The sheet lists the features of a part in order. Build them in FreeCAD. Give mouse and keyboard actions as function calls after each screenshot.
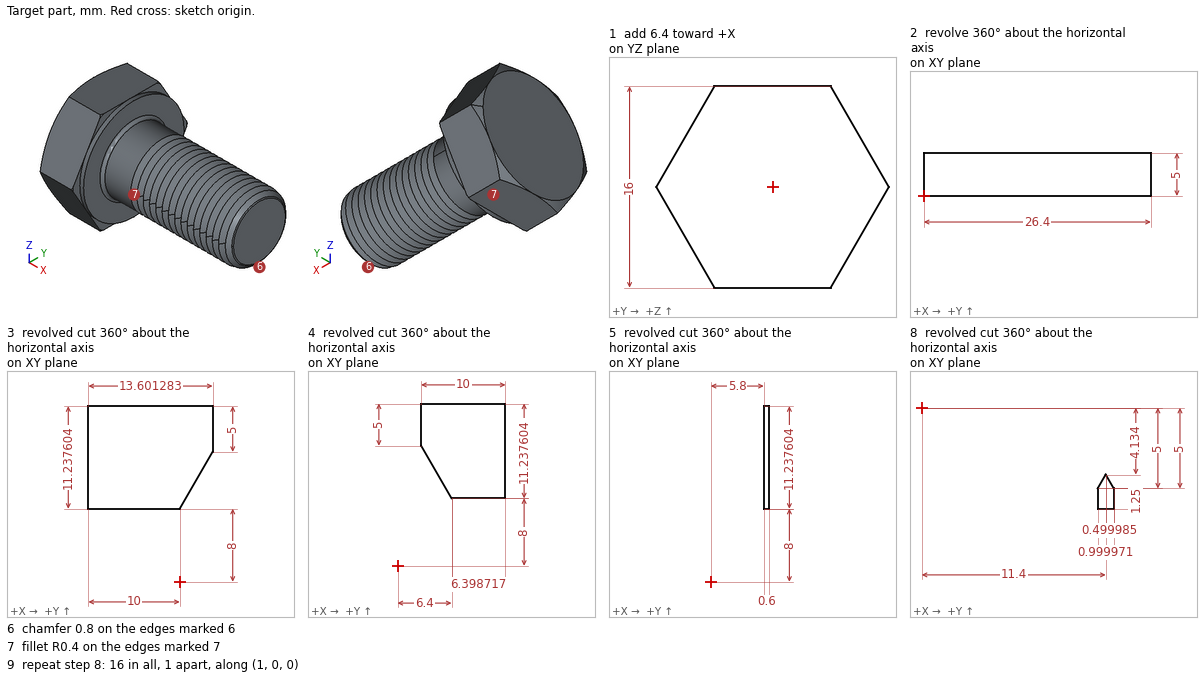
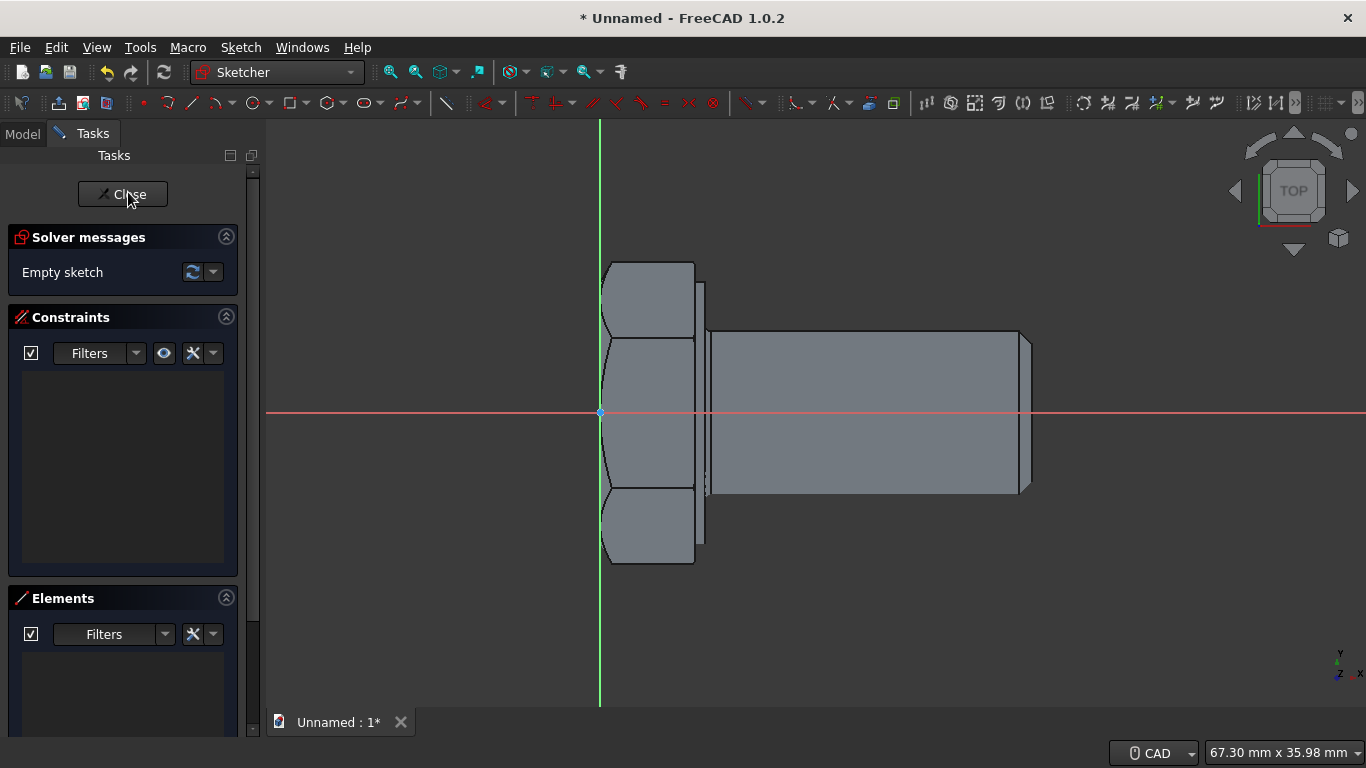
scroll(790, 506, up, 12)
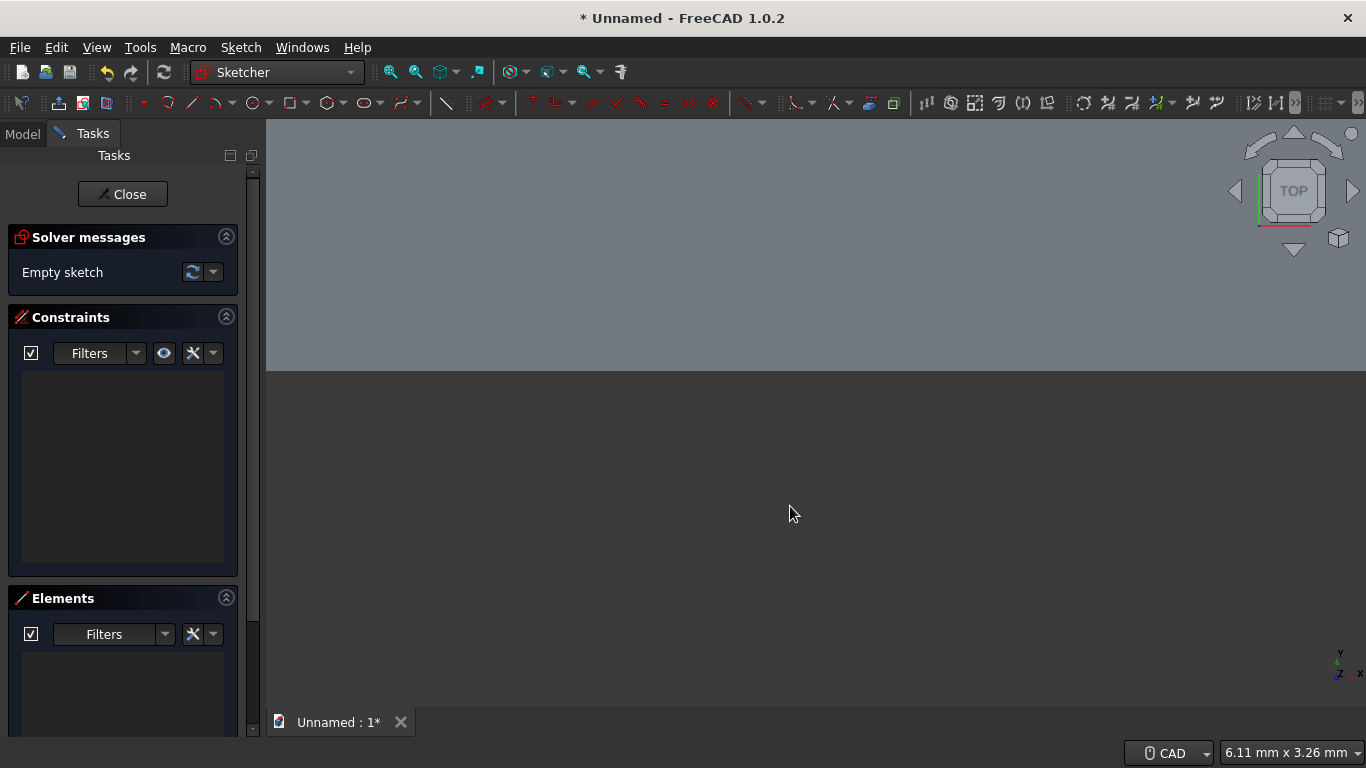
key(g)
key(m)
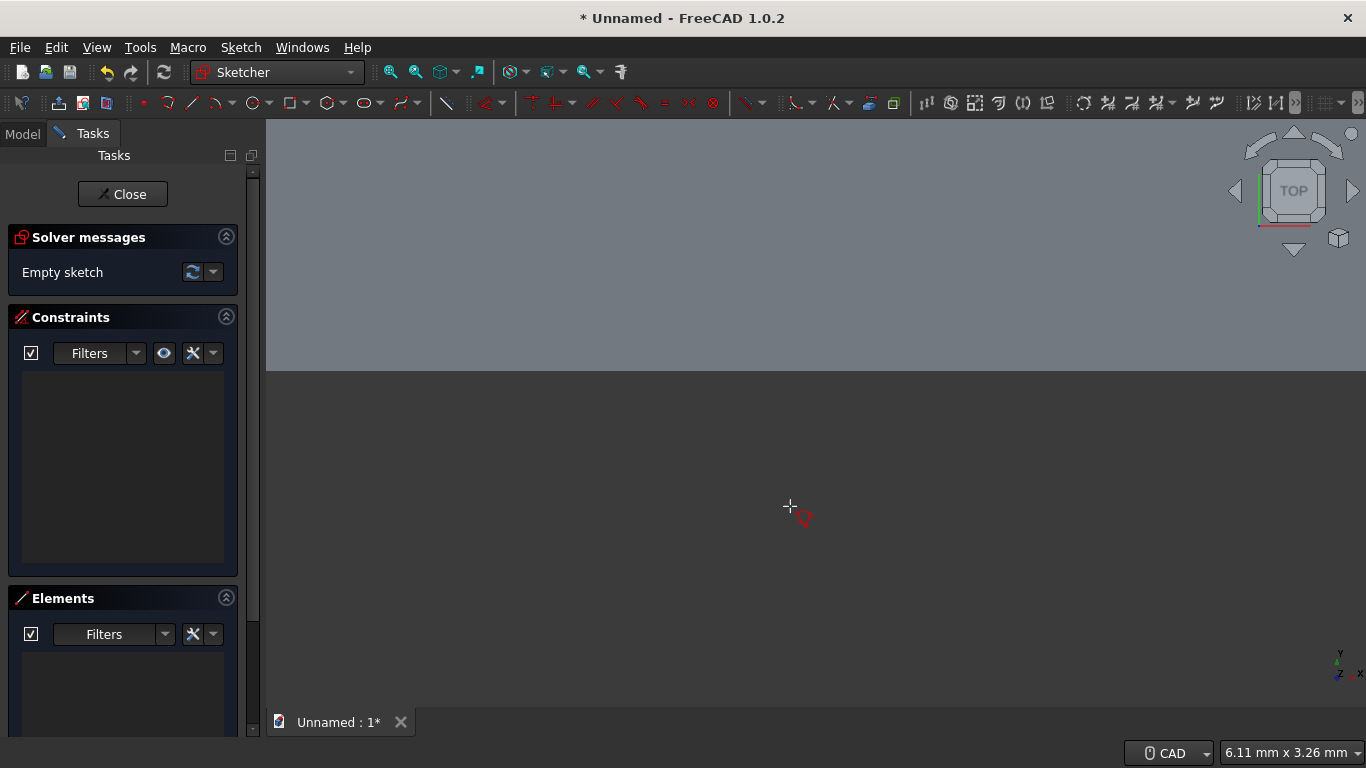
click(657, 375)
click(657, 600)
click(838, 600)
click(838, 375)
click(748, 219)
click(657, 376)
key(Escape)
key(Escape)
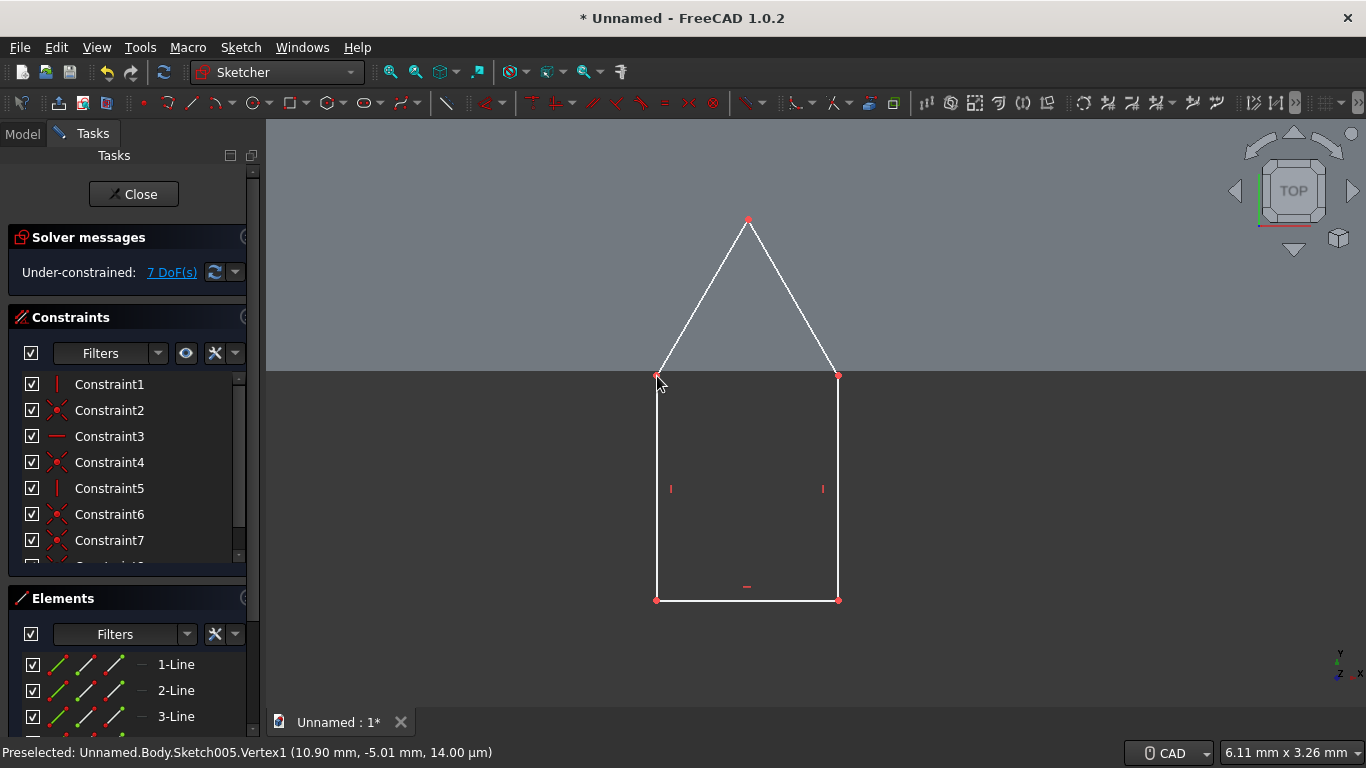
key(d)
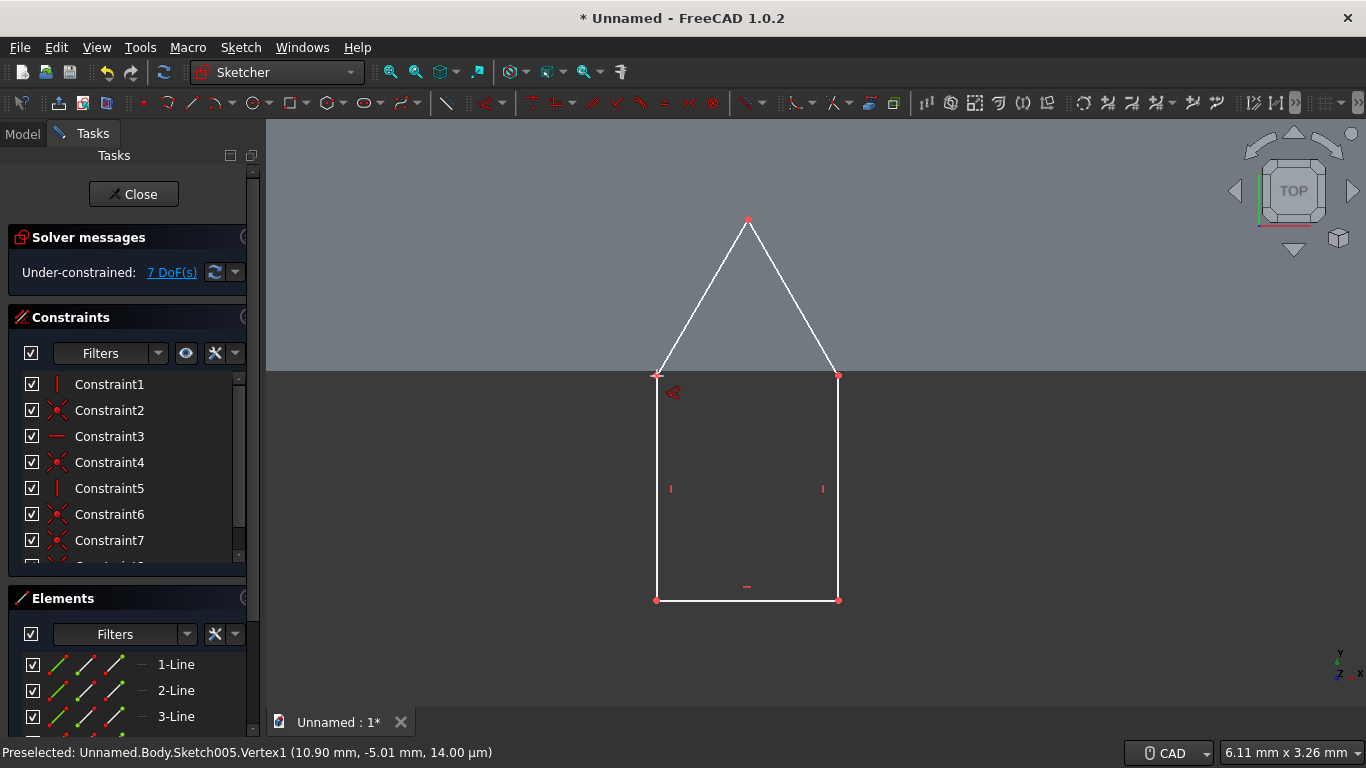
click(657, 376)
click(691, 262)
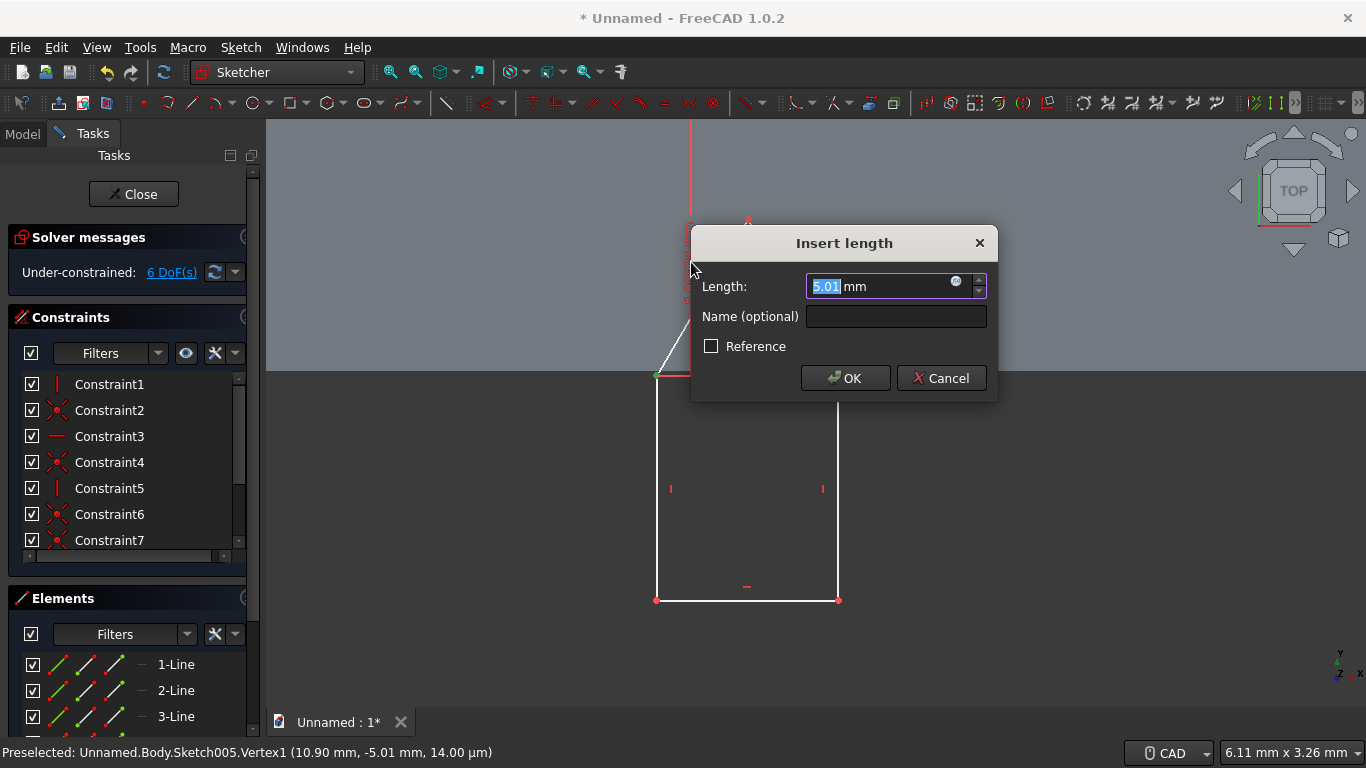
text(5)
key(Return)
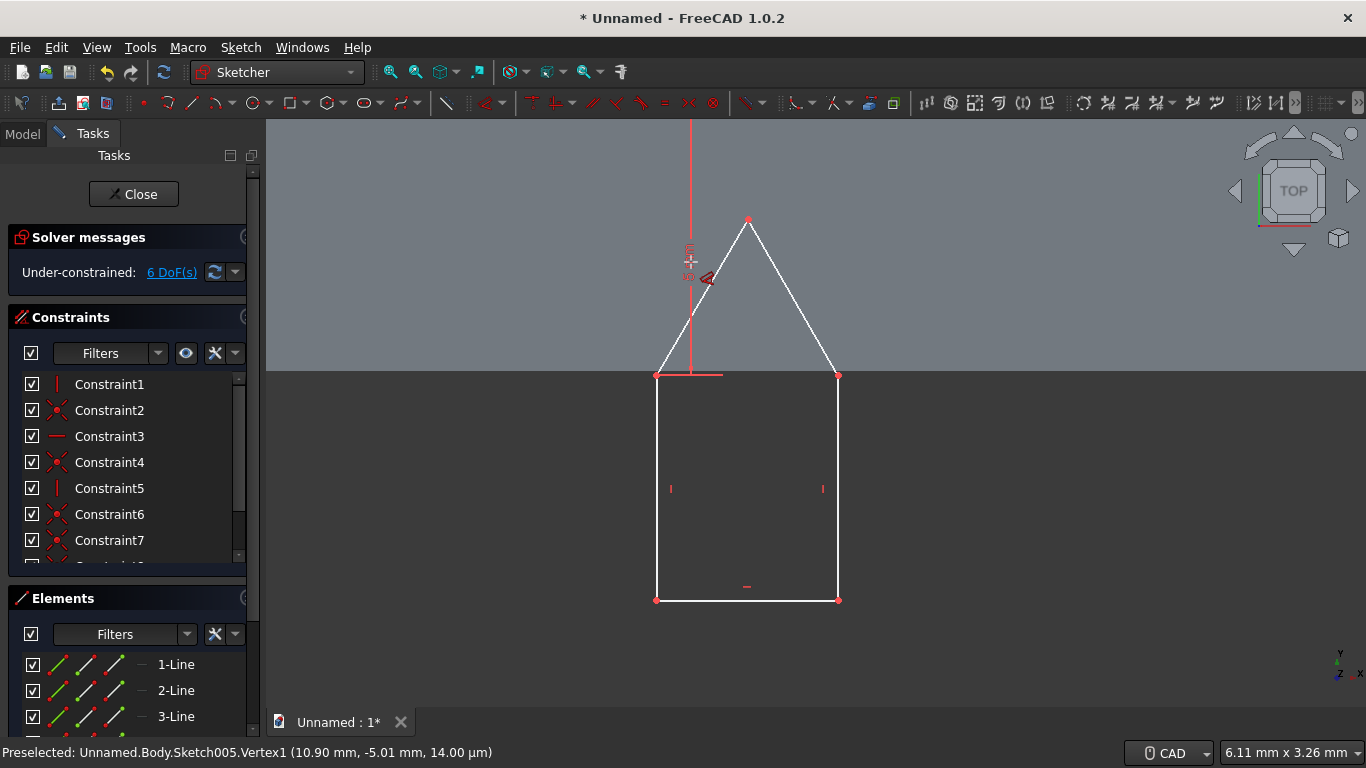
click(838, 376)
click(872, 262)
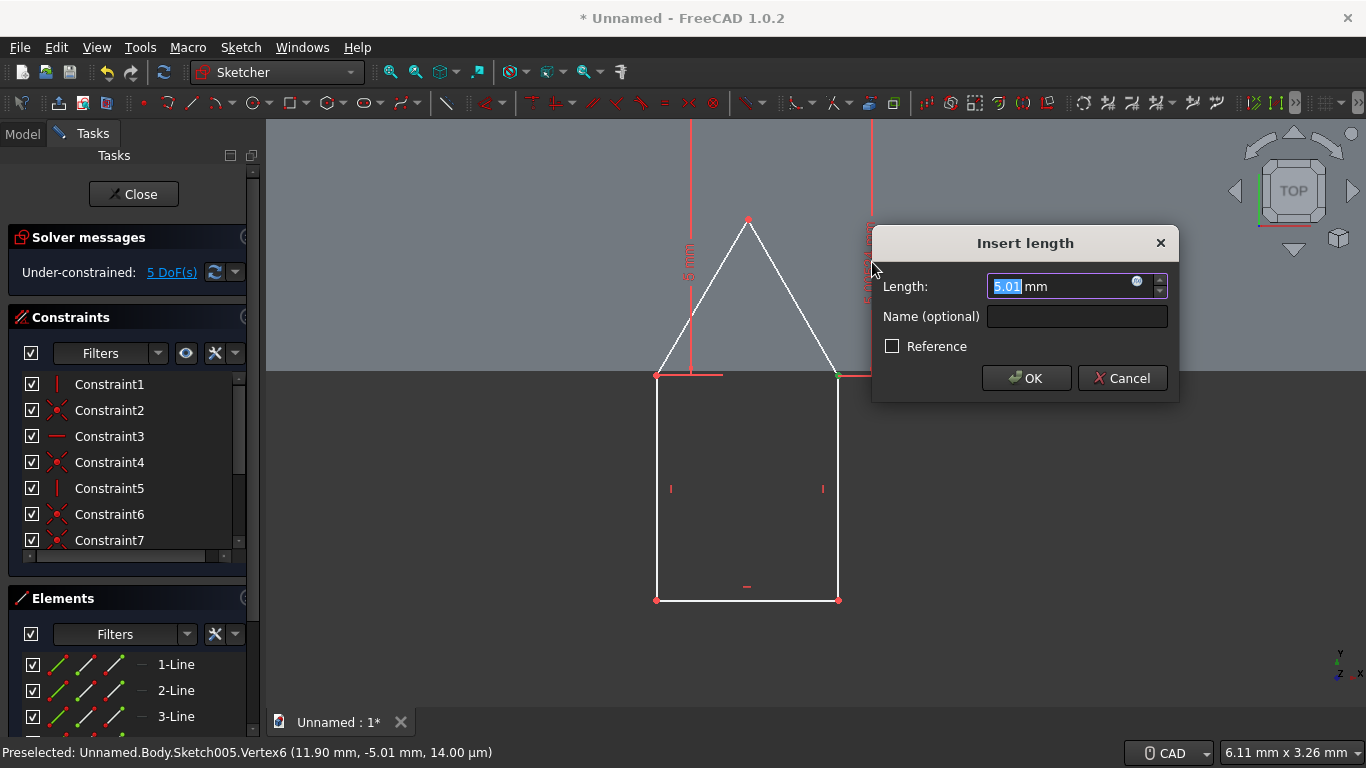
text(5)
key(Return)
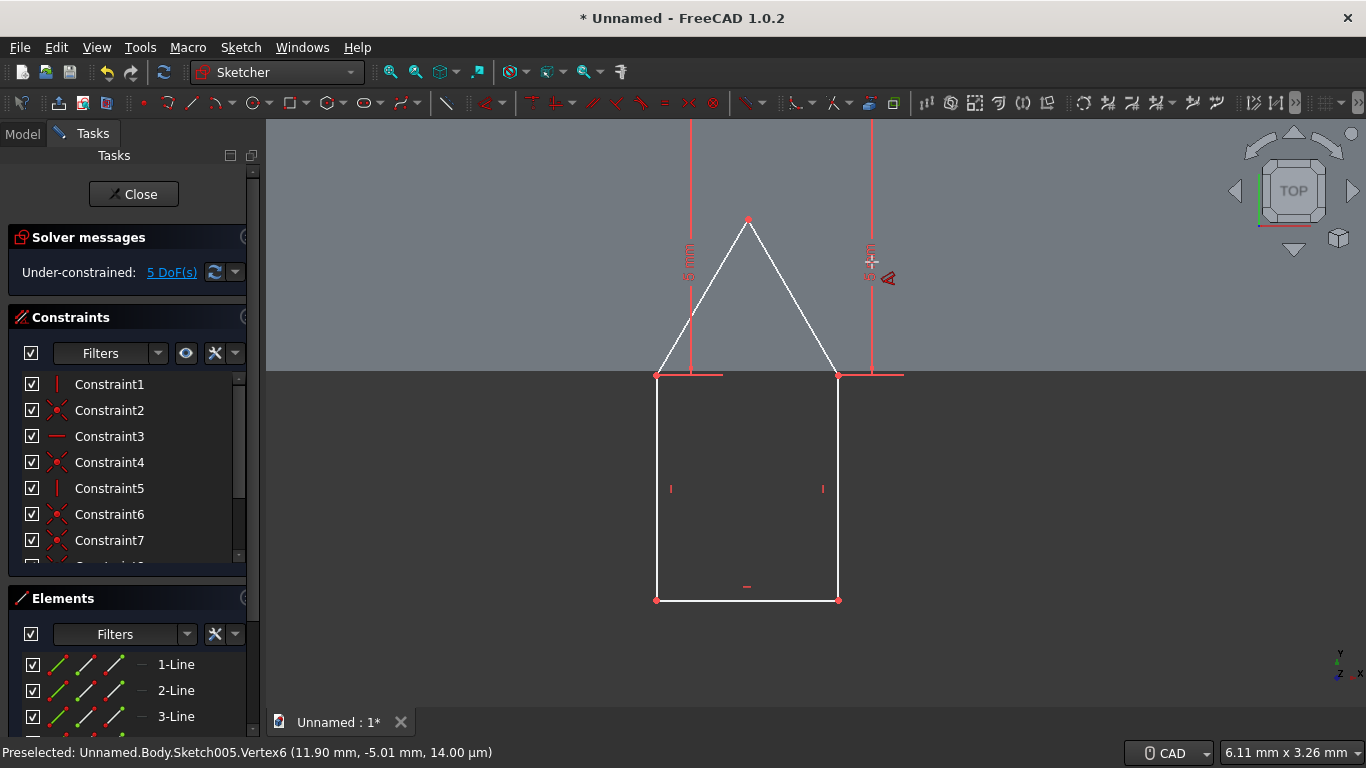
click(657, 443)
click(623, 488)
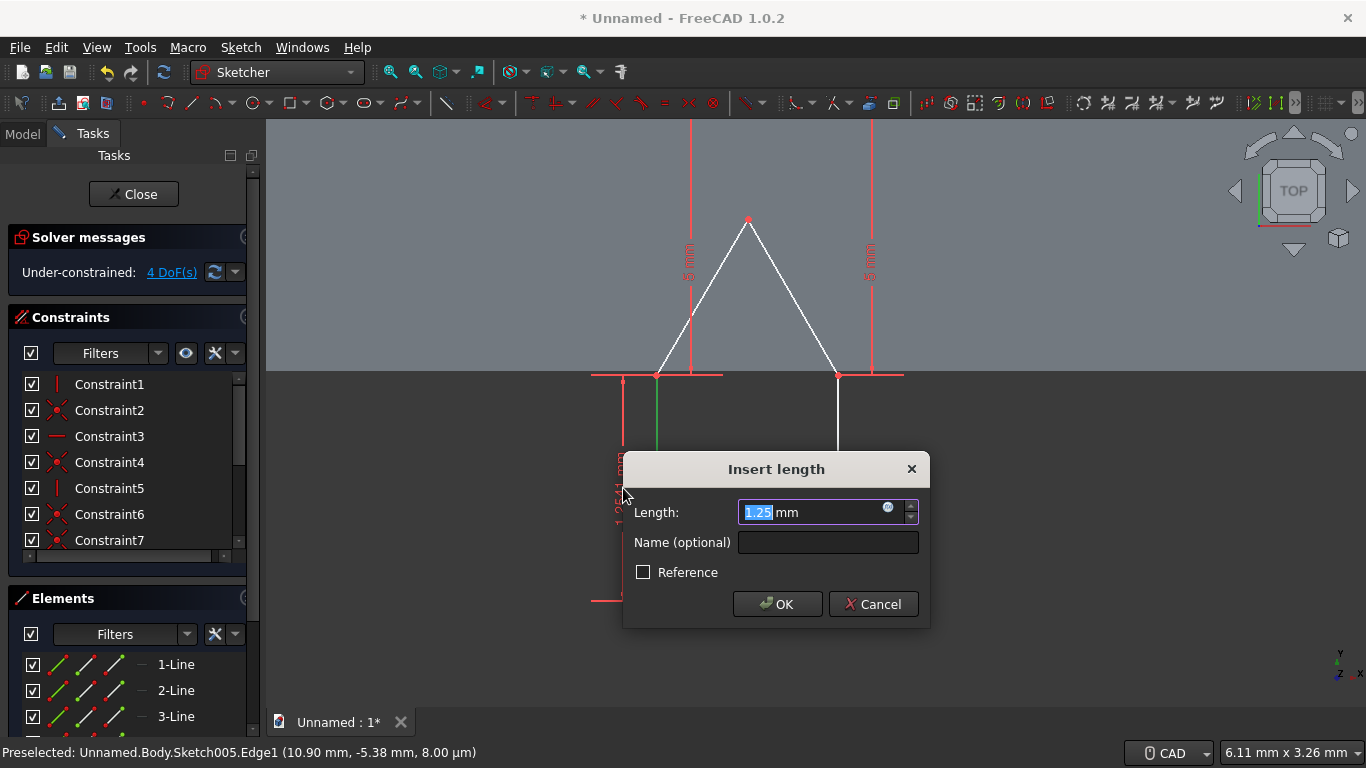
text(1.25)
key(Return)